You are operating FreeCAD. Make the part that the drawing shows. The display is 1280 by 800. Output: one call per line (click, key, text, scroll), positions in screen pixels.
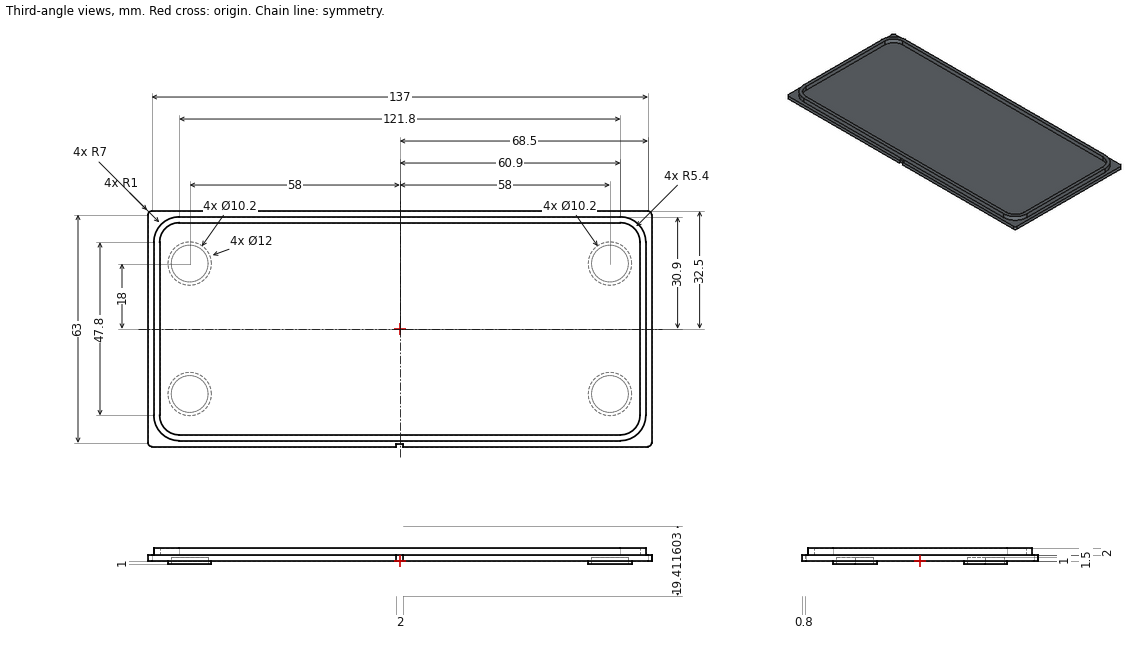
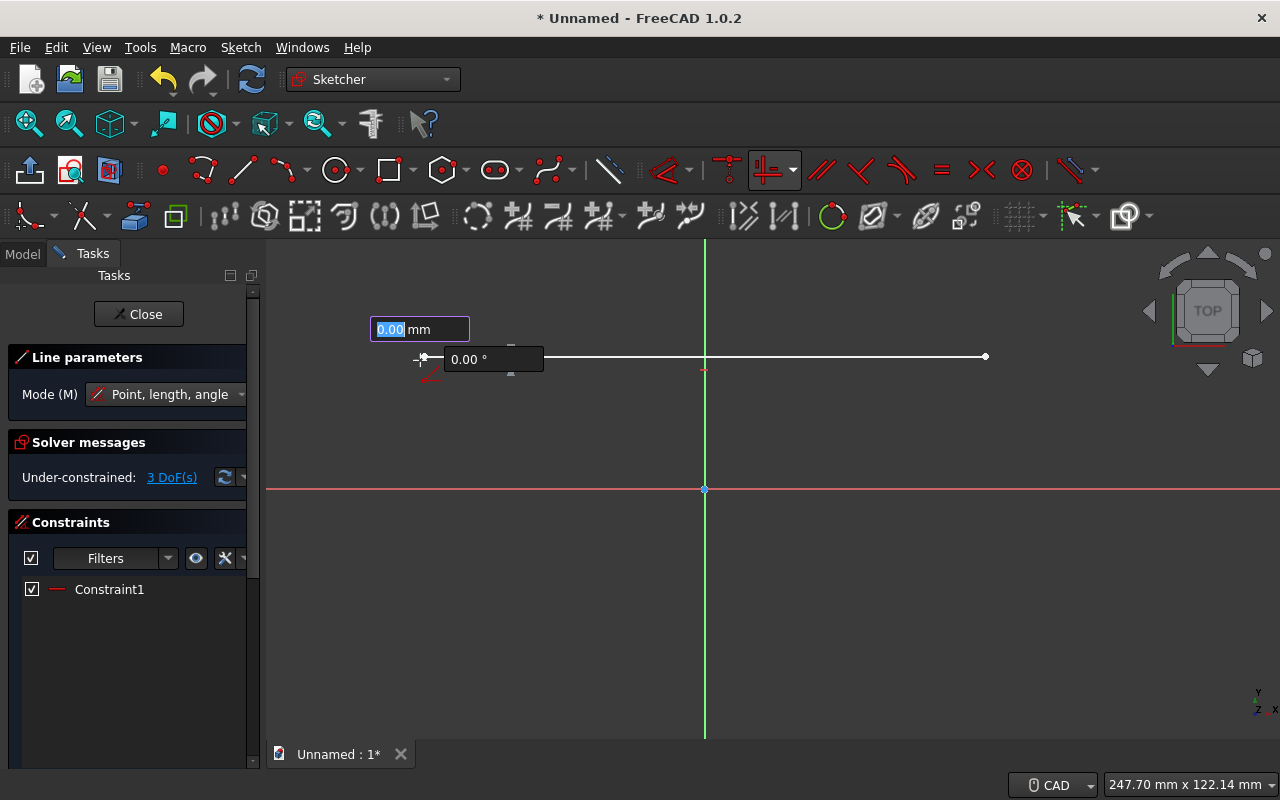
click(420, 618)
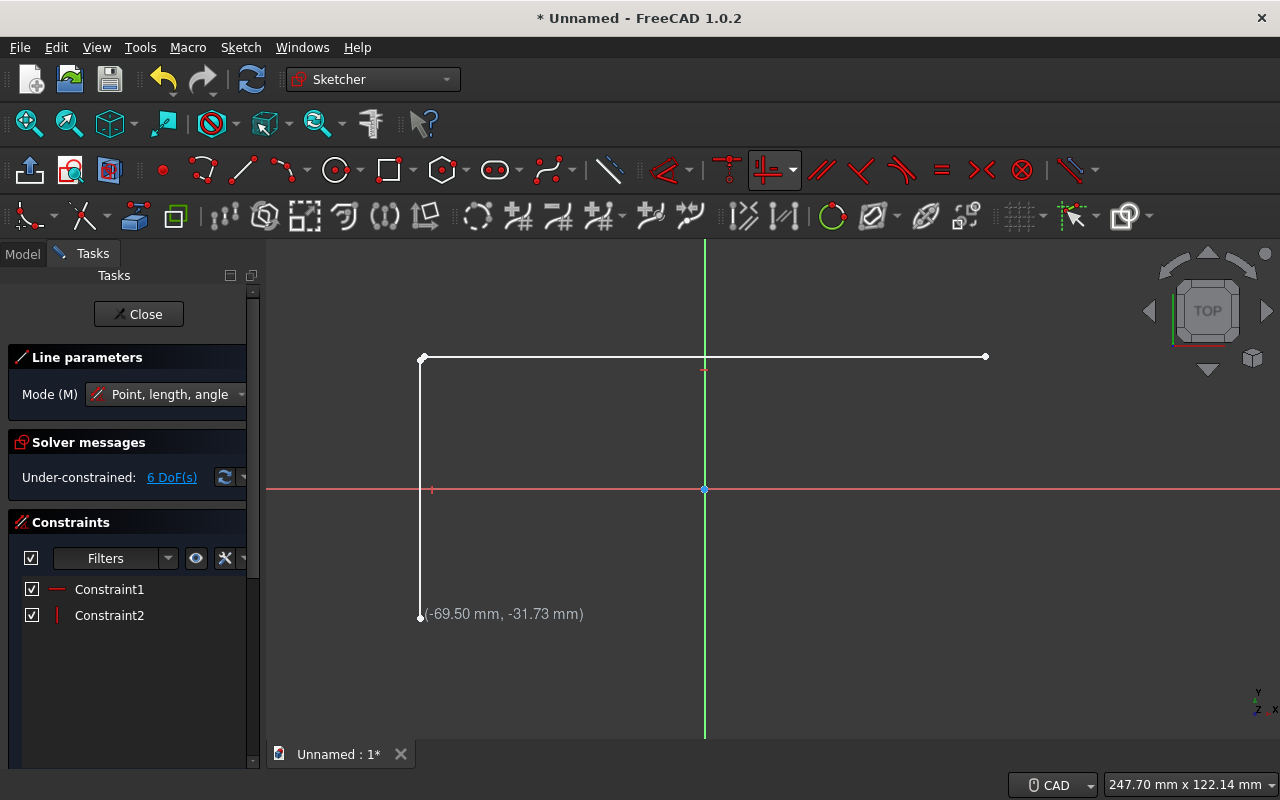
scroll(424, 622, up, 6)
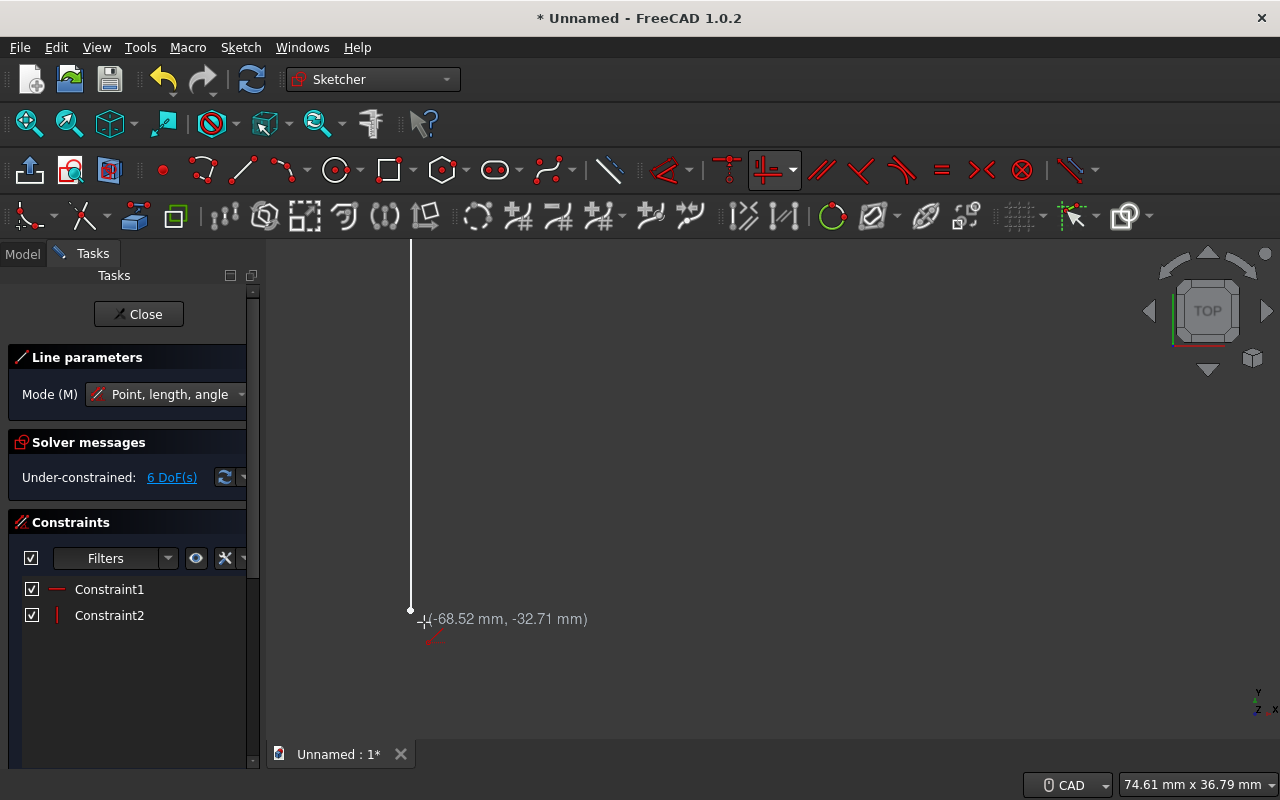
click(424, 621)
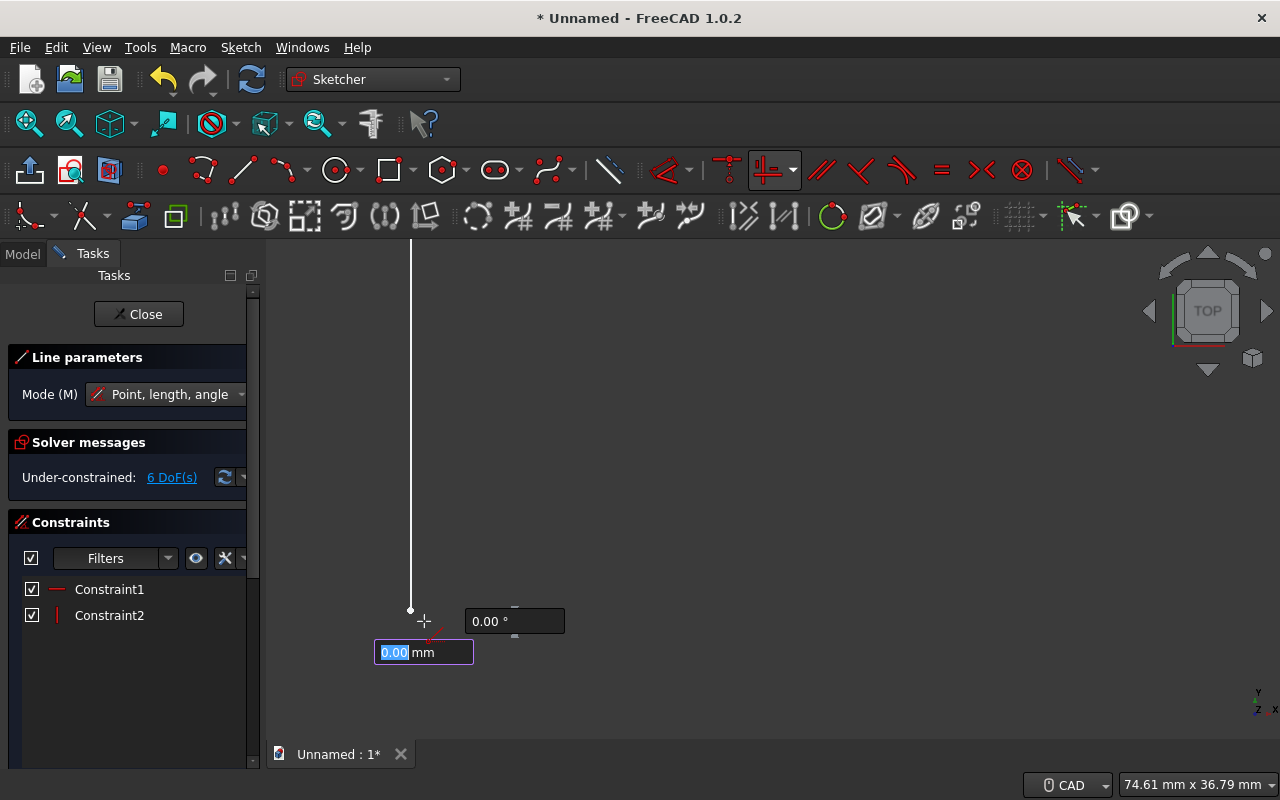
scroll(424, 623, down, 6)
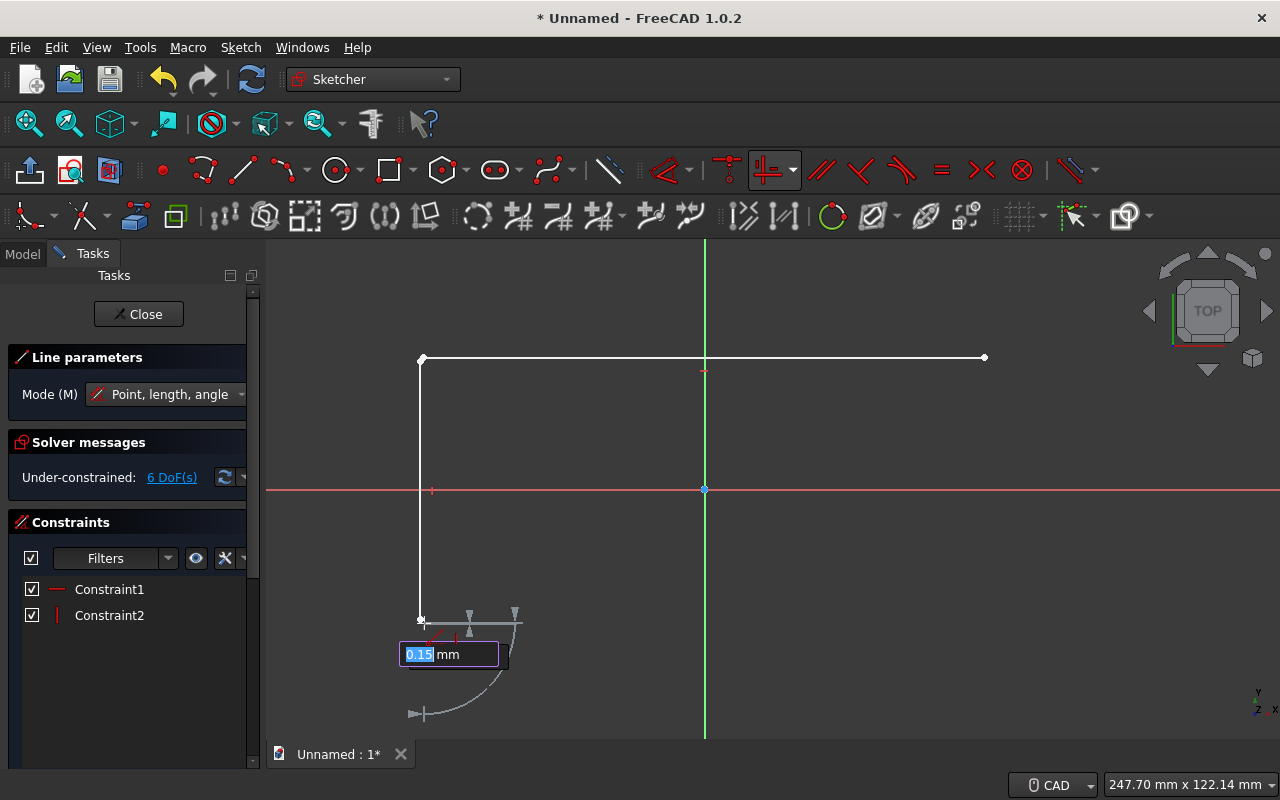
click(985, 623)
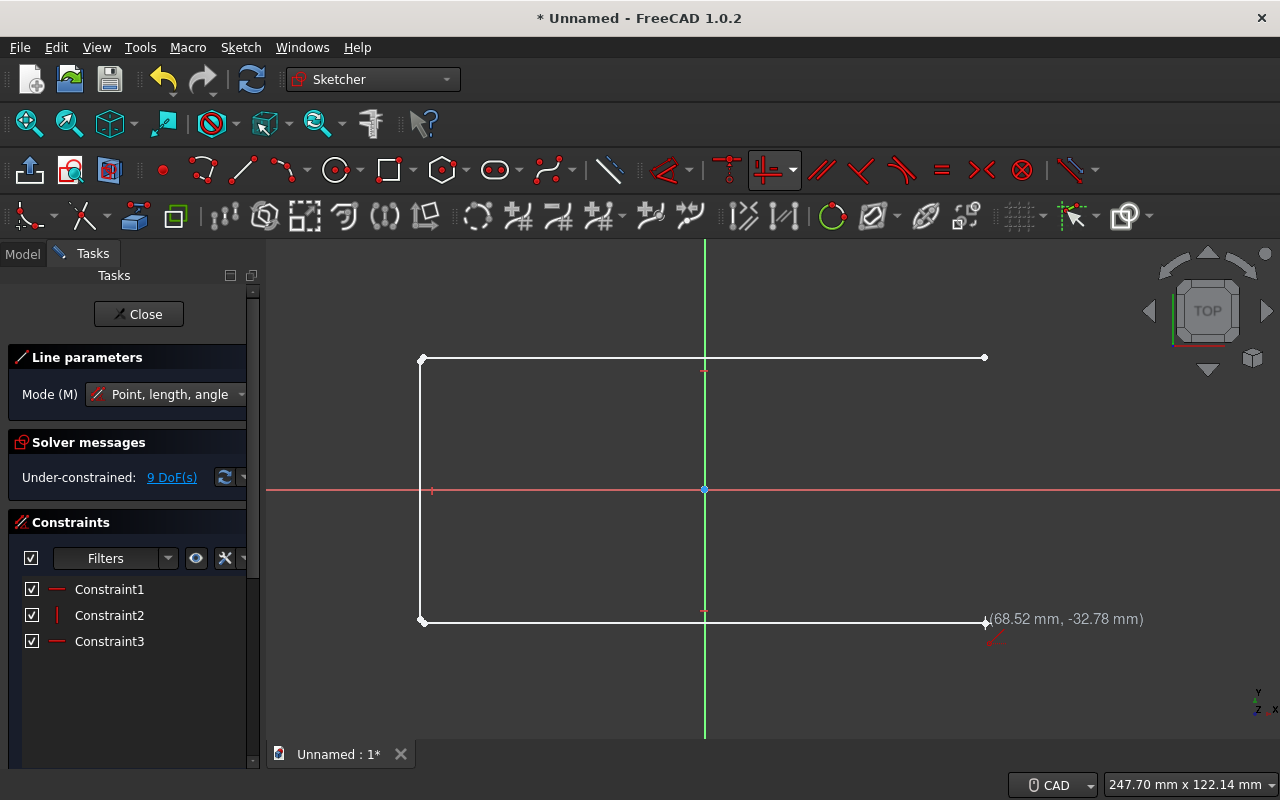
scroll(989, 619, up, 6)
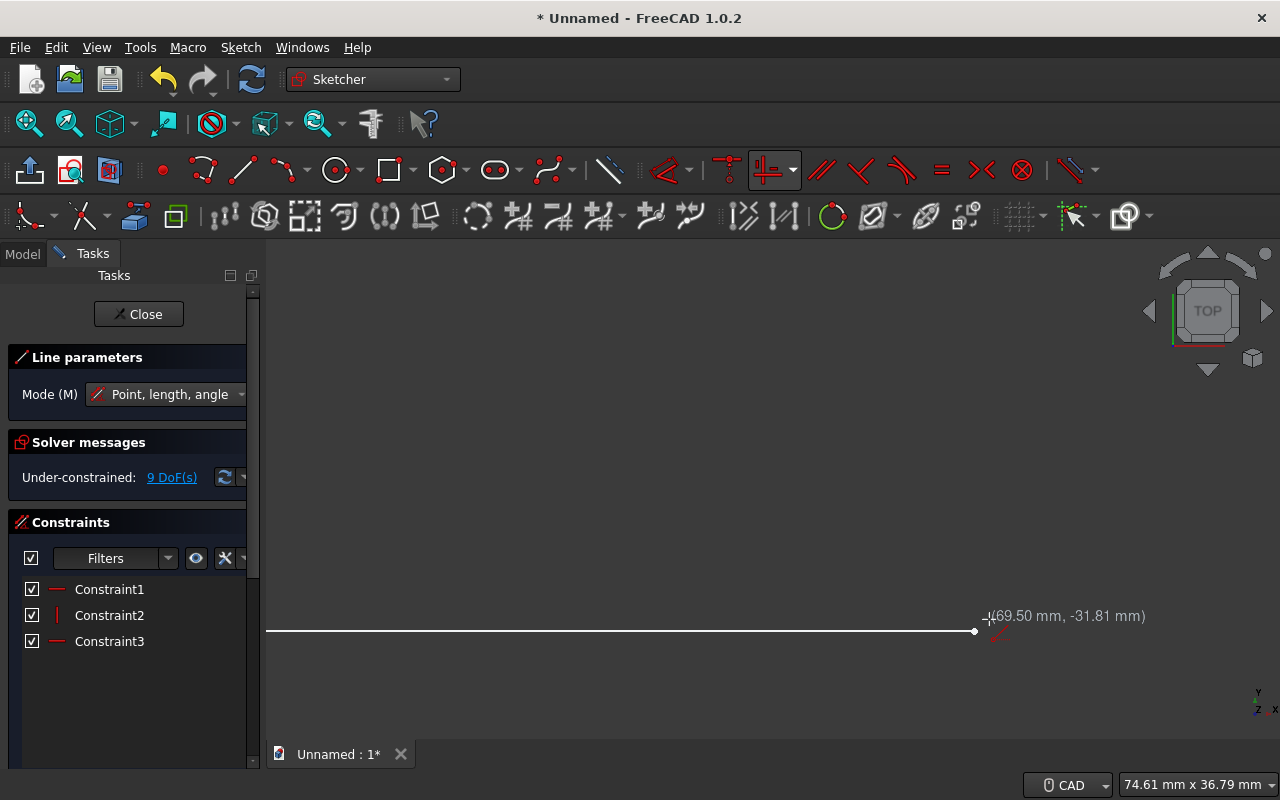
click(987, 616)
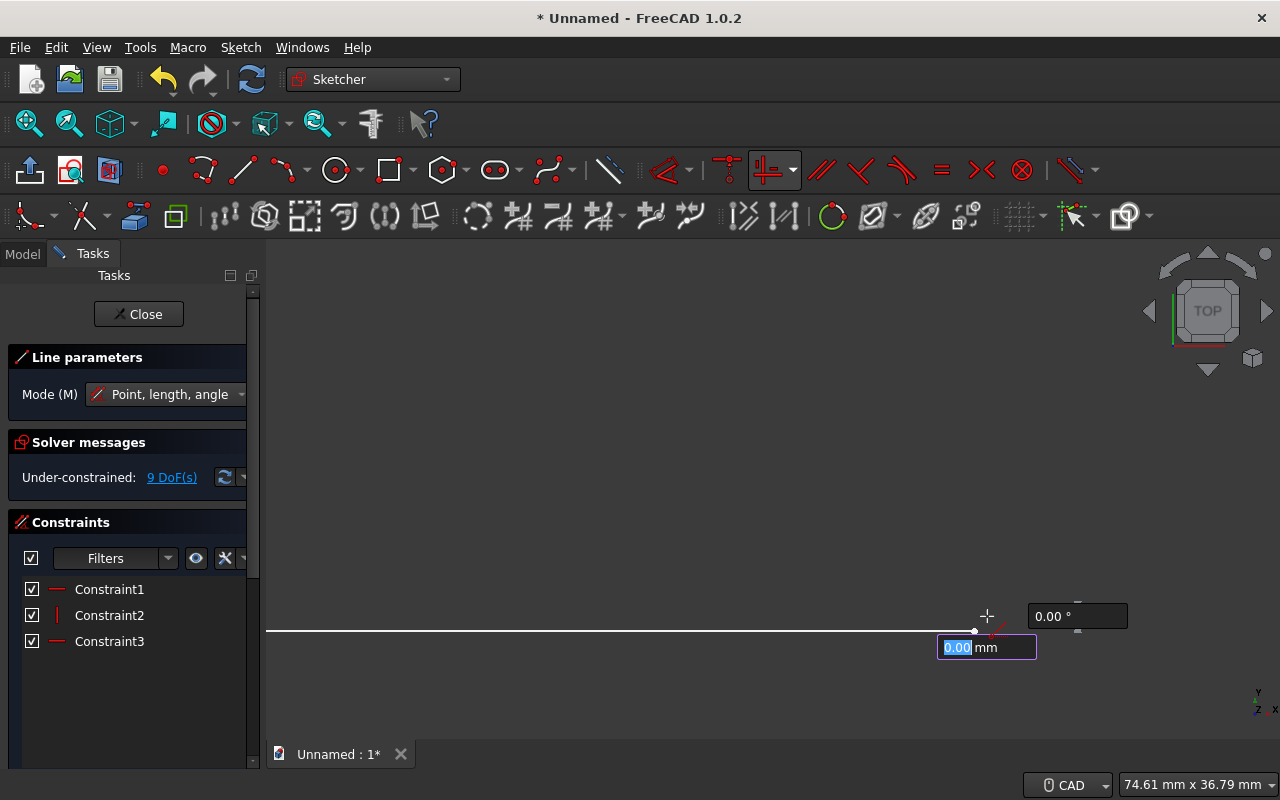
scroll(990, 619, down, 6)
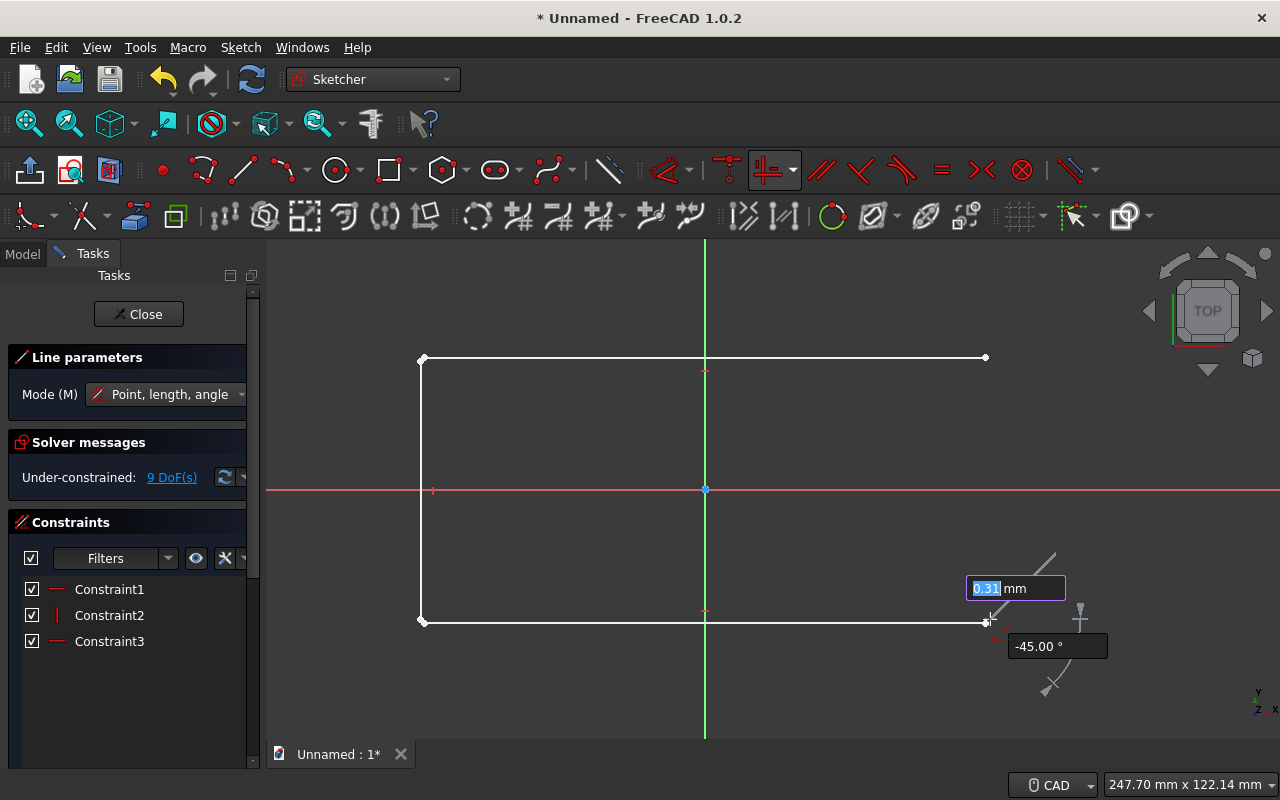
scroll(990, 361, up, 6)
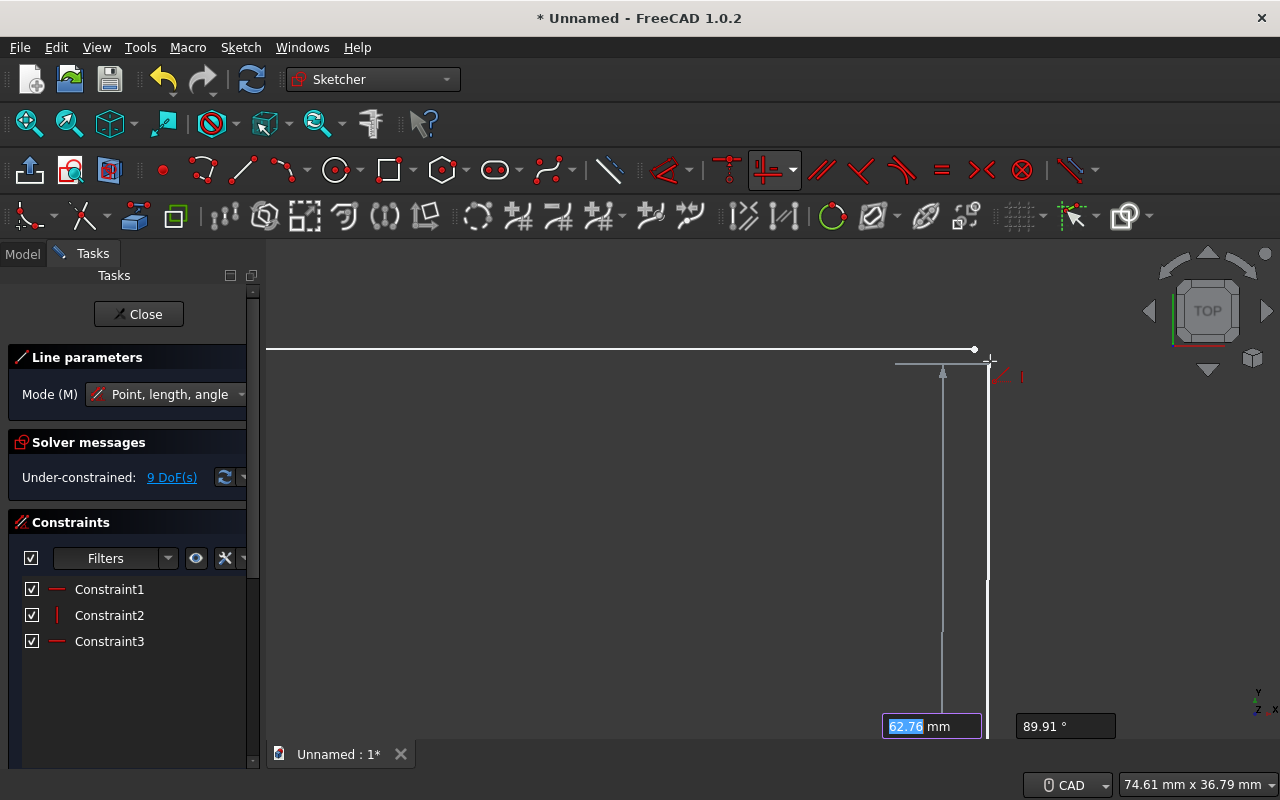
click(987, 360)